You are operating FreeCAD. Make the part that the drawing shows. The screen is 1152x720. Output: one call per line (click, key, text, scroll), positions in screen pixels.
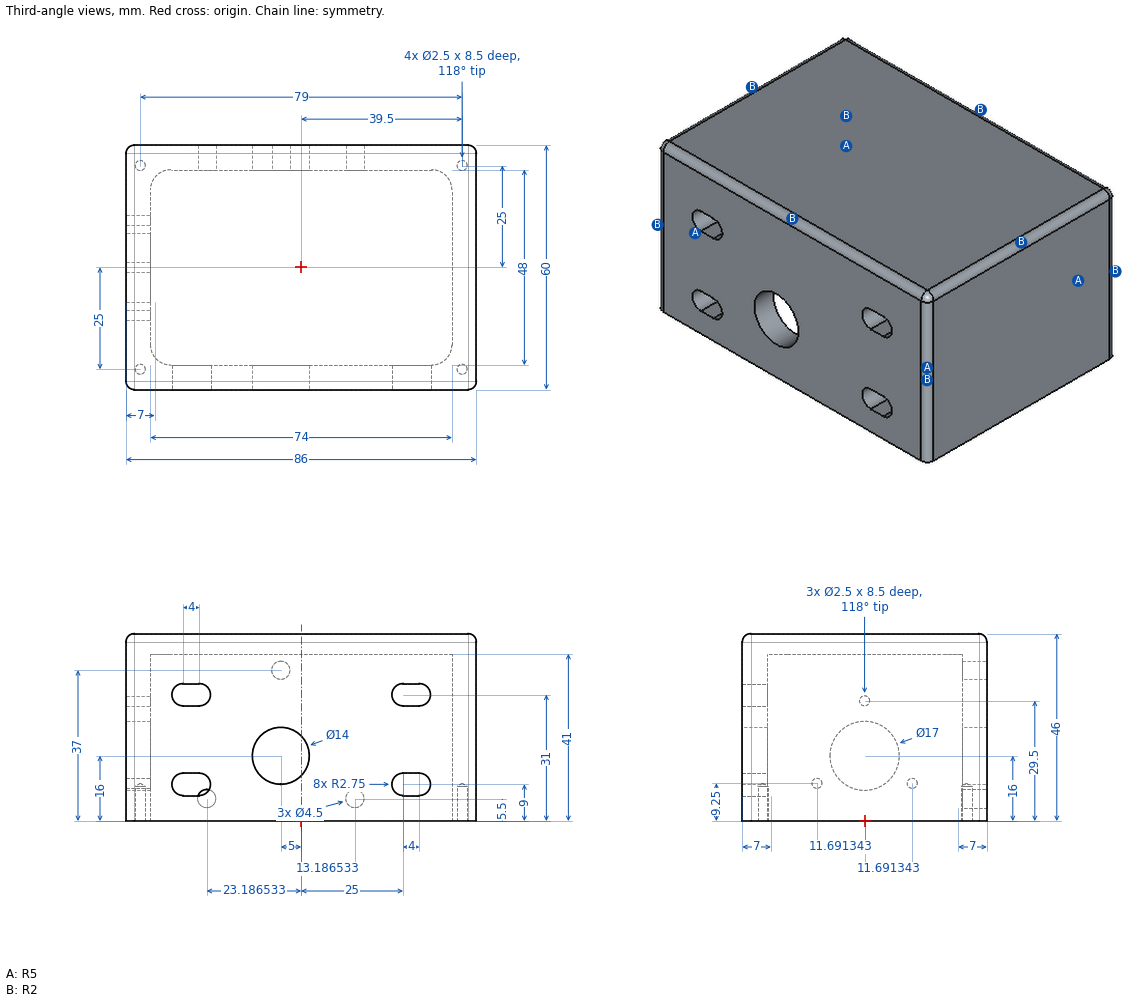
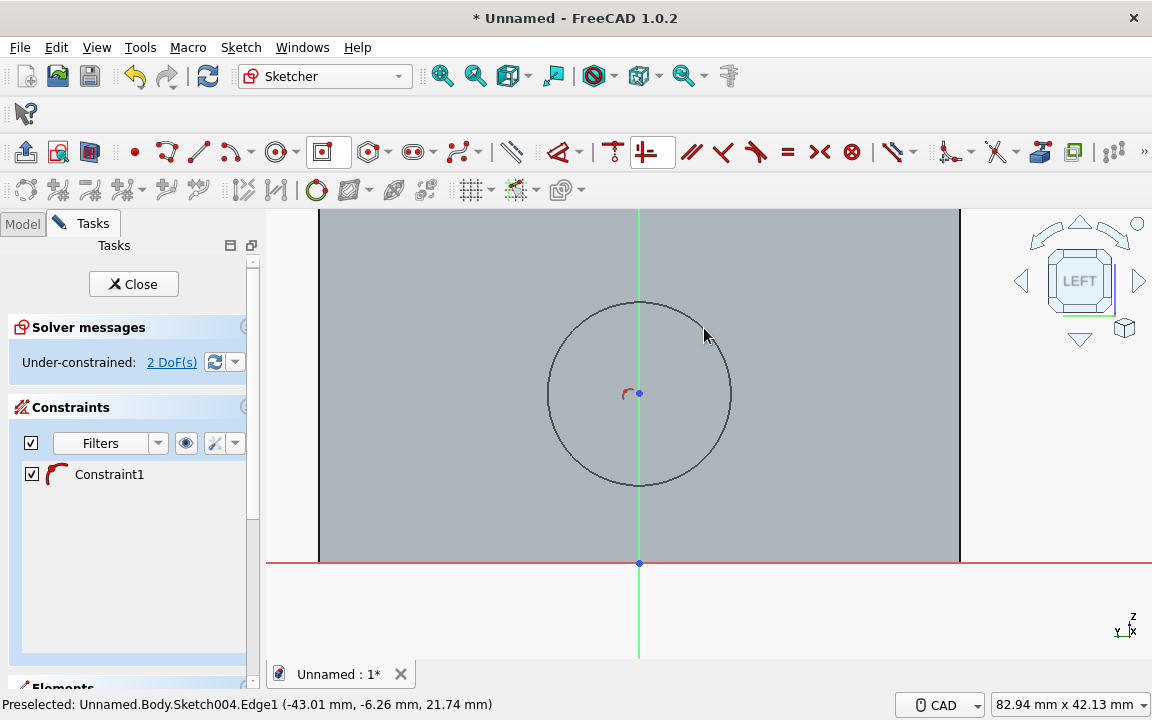
key(d)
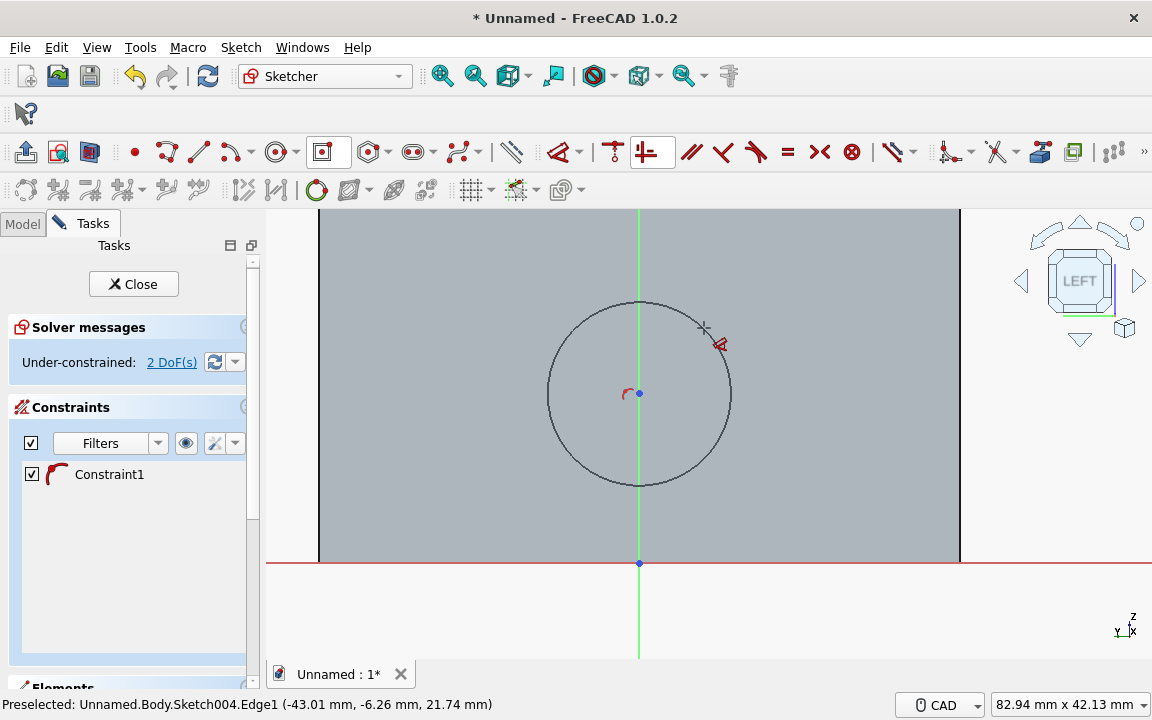
click(704, 329)
click(727, 306)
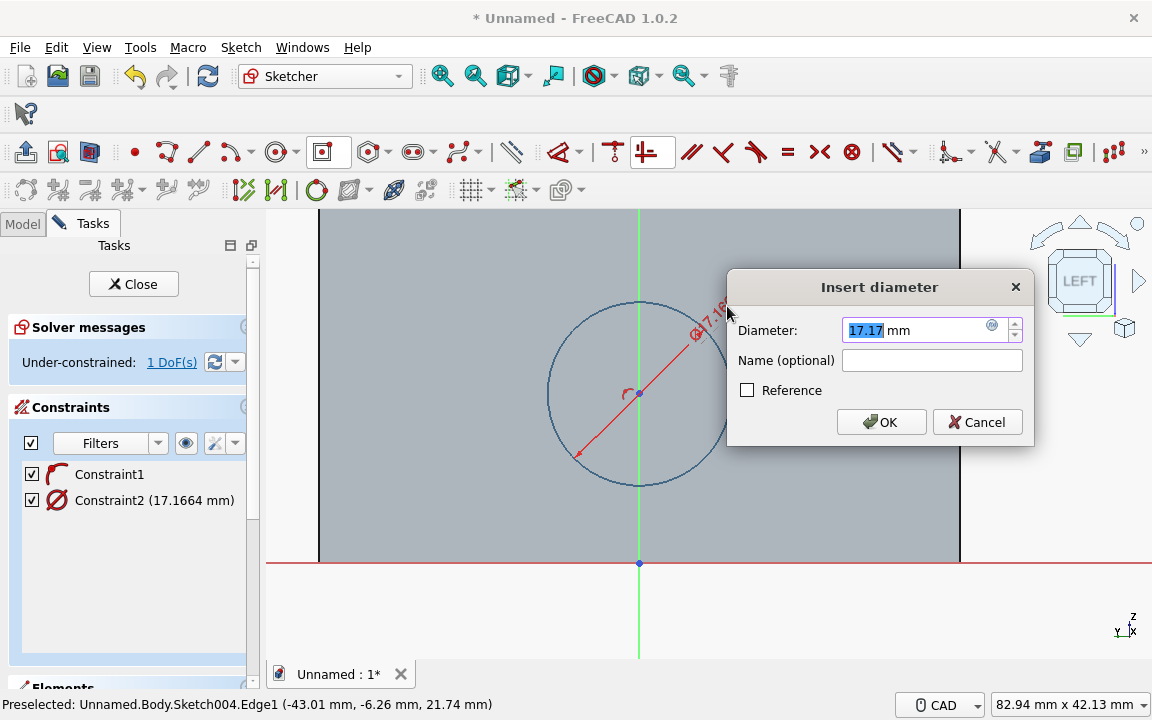
text(17)
key(Return)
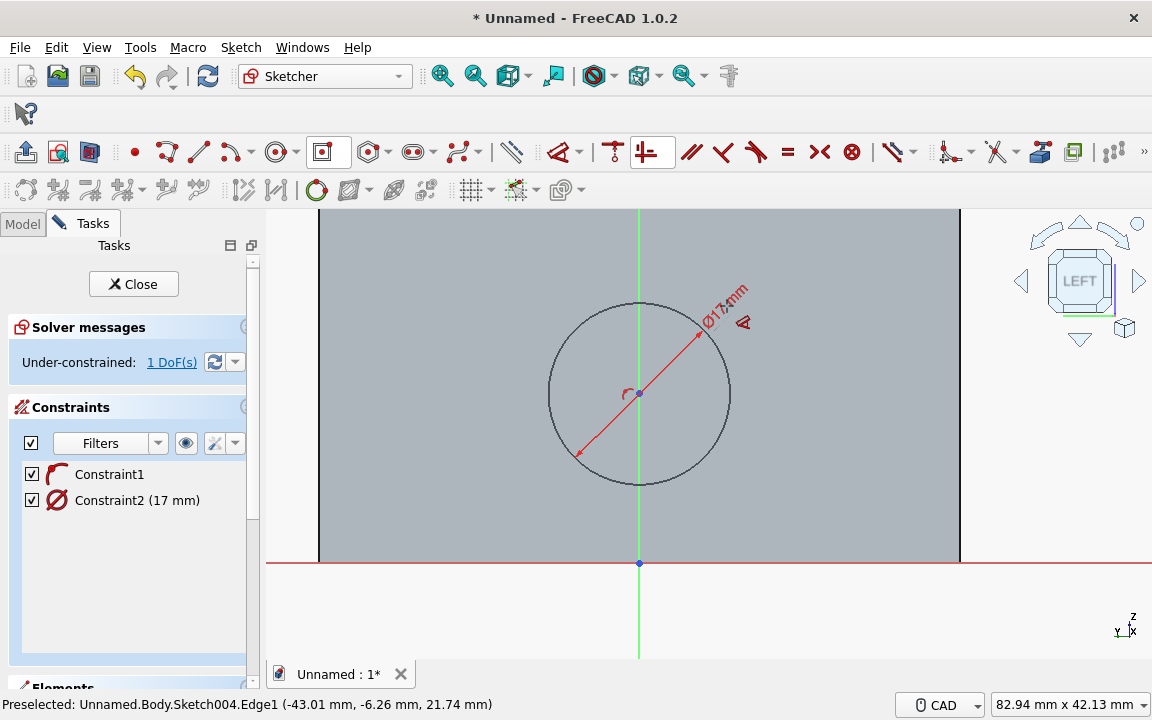
click(639, 394)
click(673, 440)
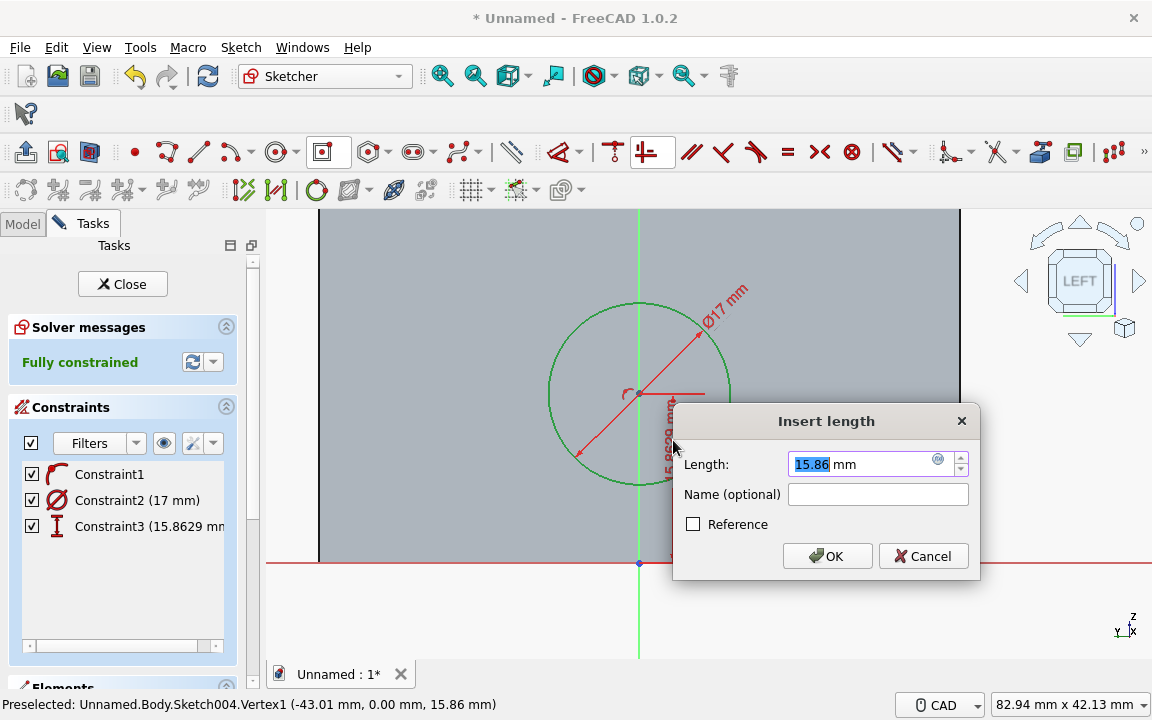
text(16)
key(Return)
key(Escape)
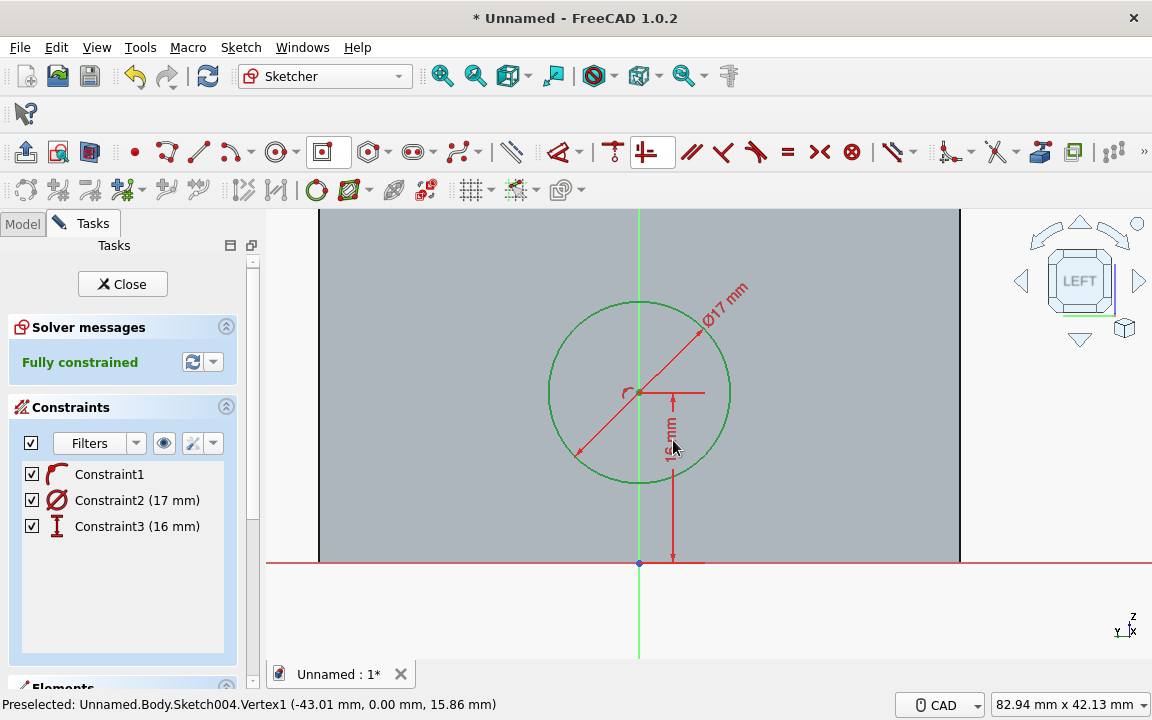
click(123, 284)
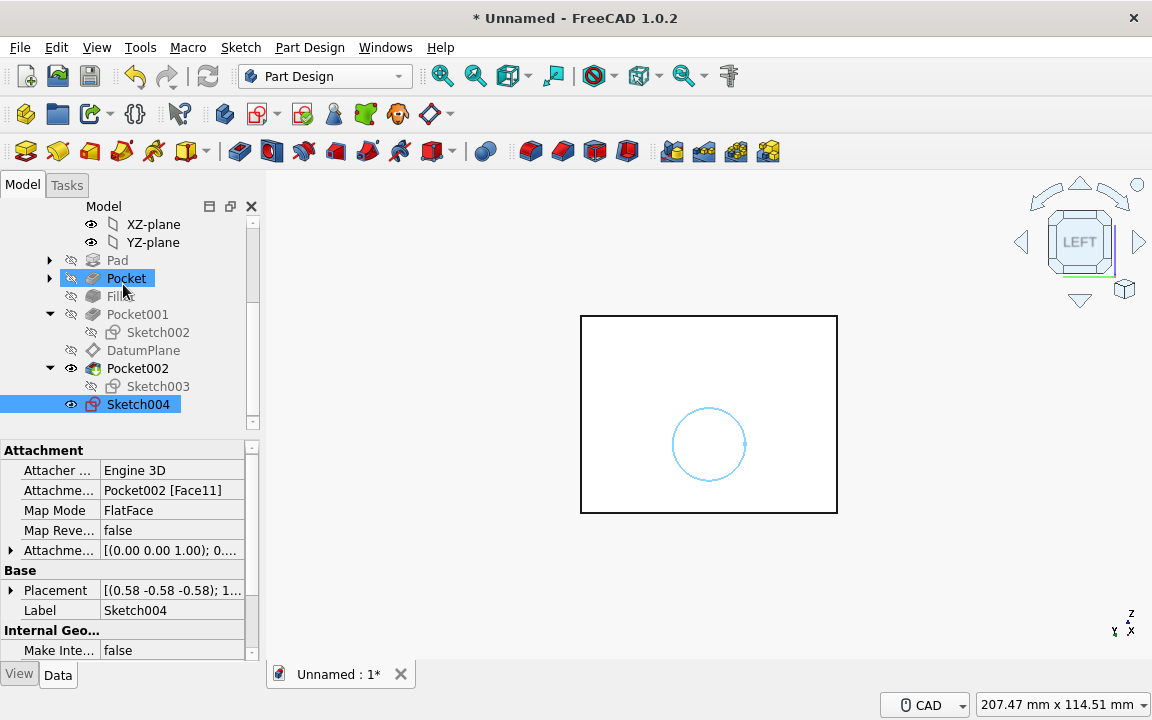
click(240, 152)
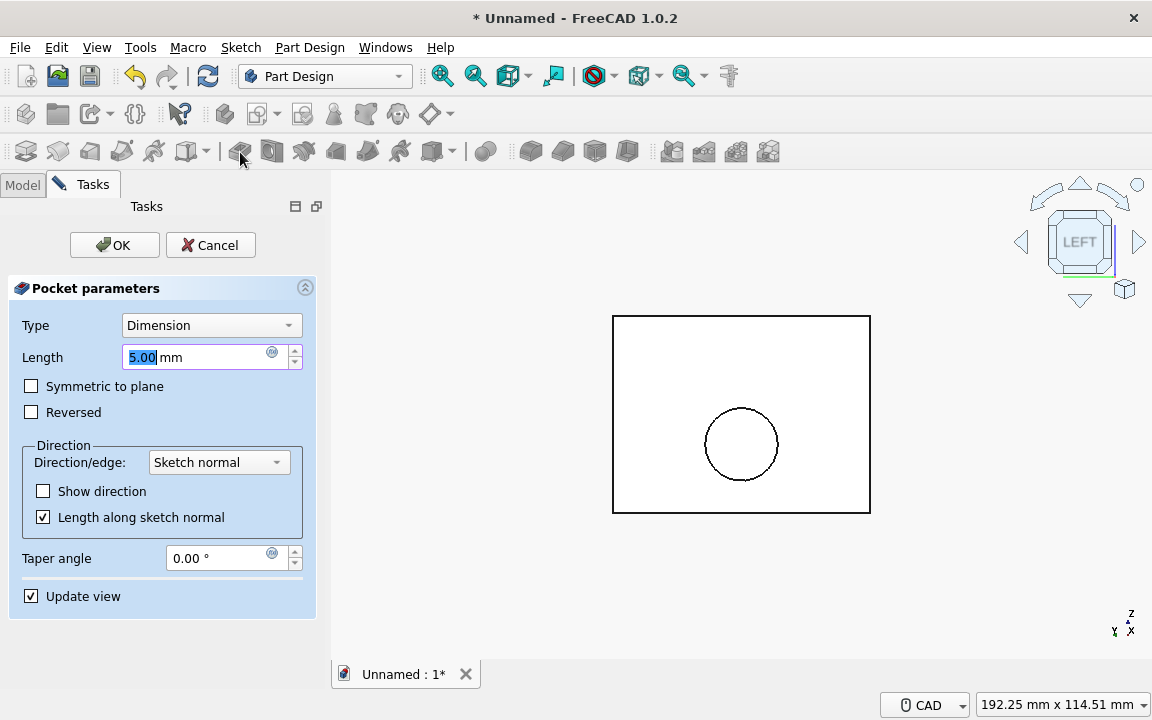
text(7)
key(Tab)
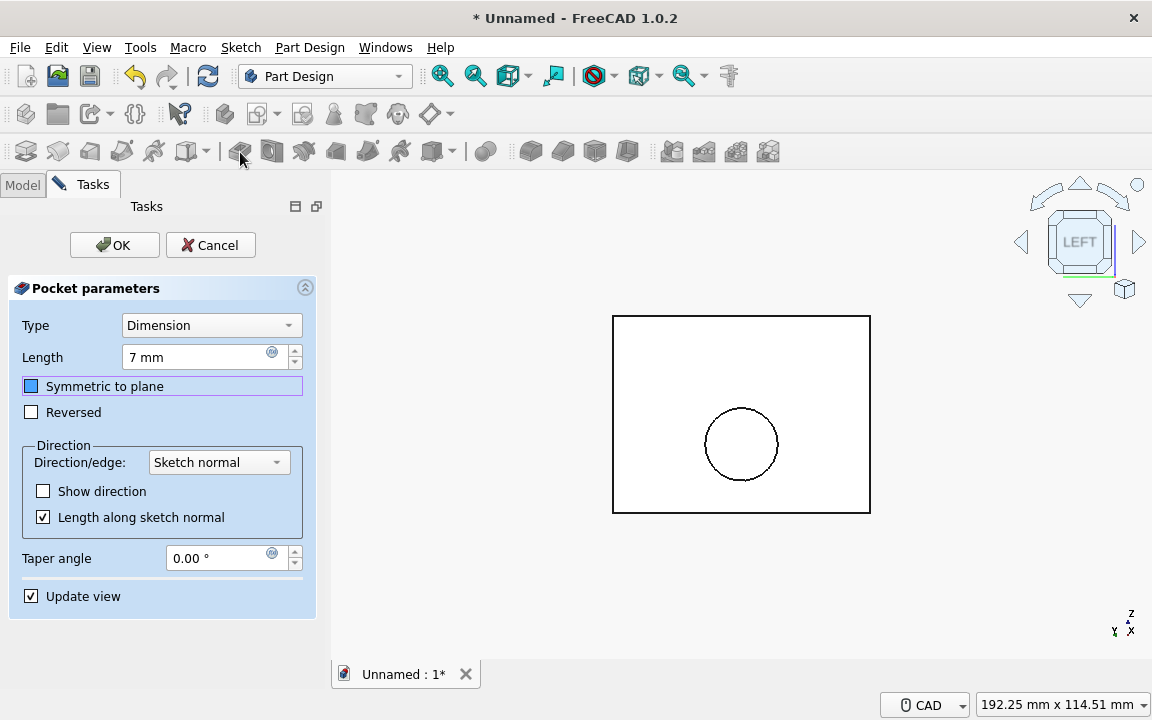
click(115, 245)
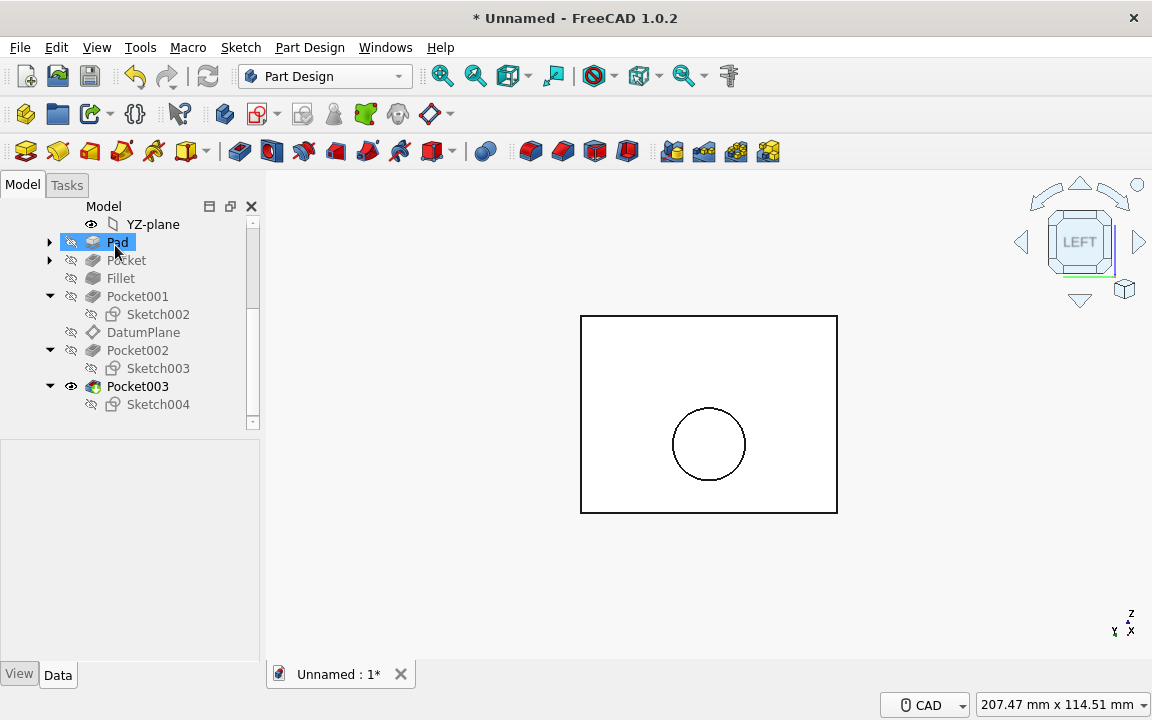
click(444, 76)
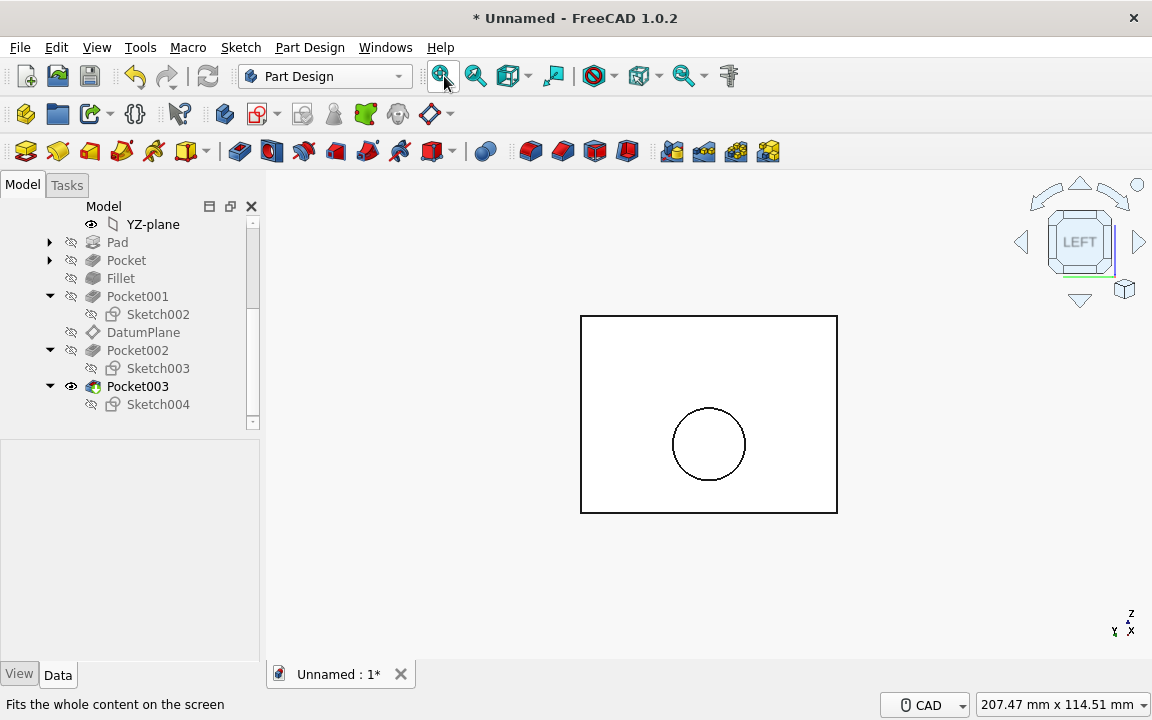
click(636, 385)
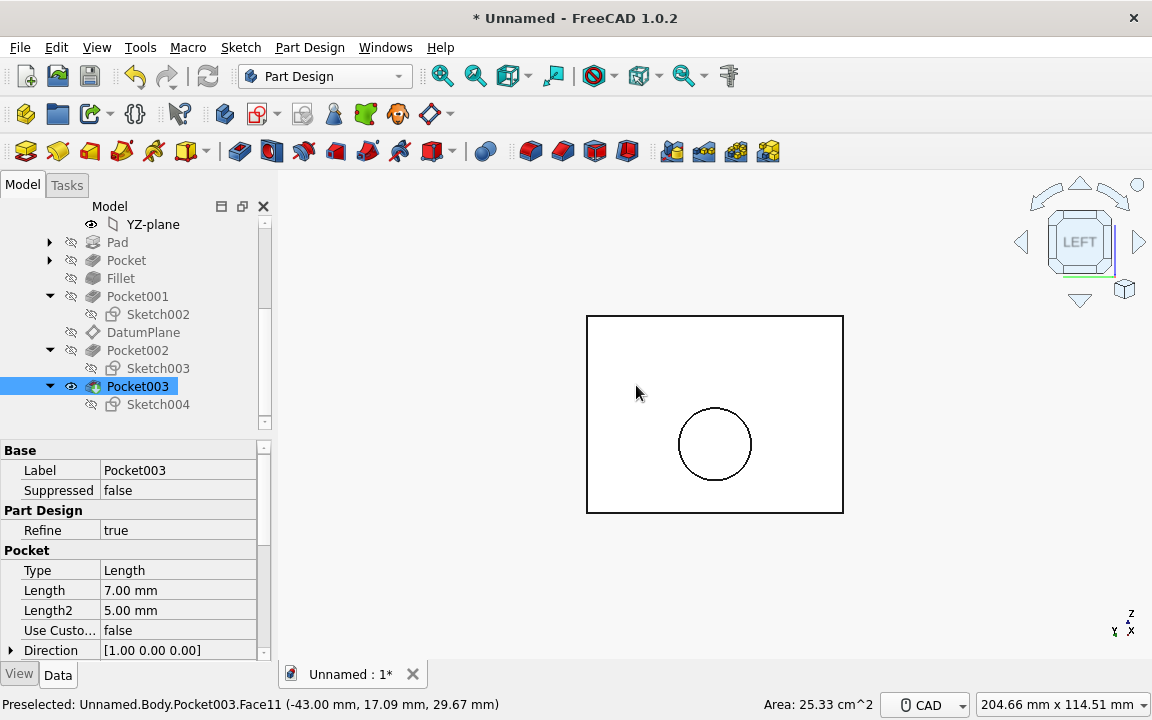
click(258, 114)